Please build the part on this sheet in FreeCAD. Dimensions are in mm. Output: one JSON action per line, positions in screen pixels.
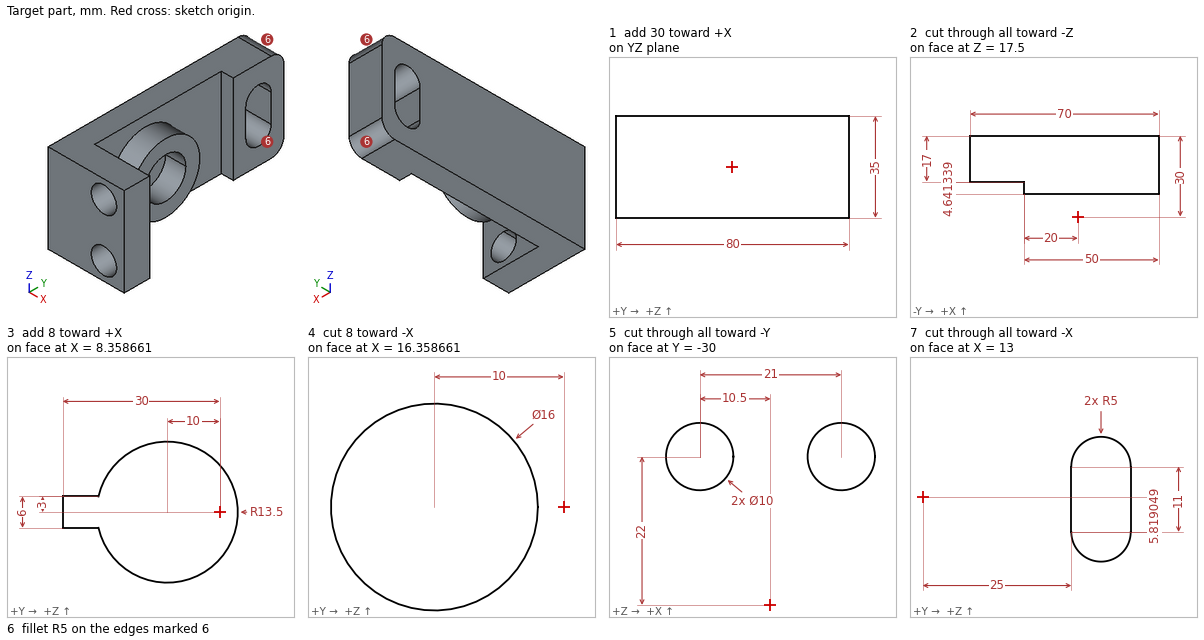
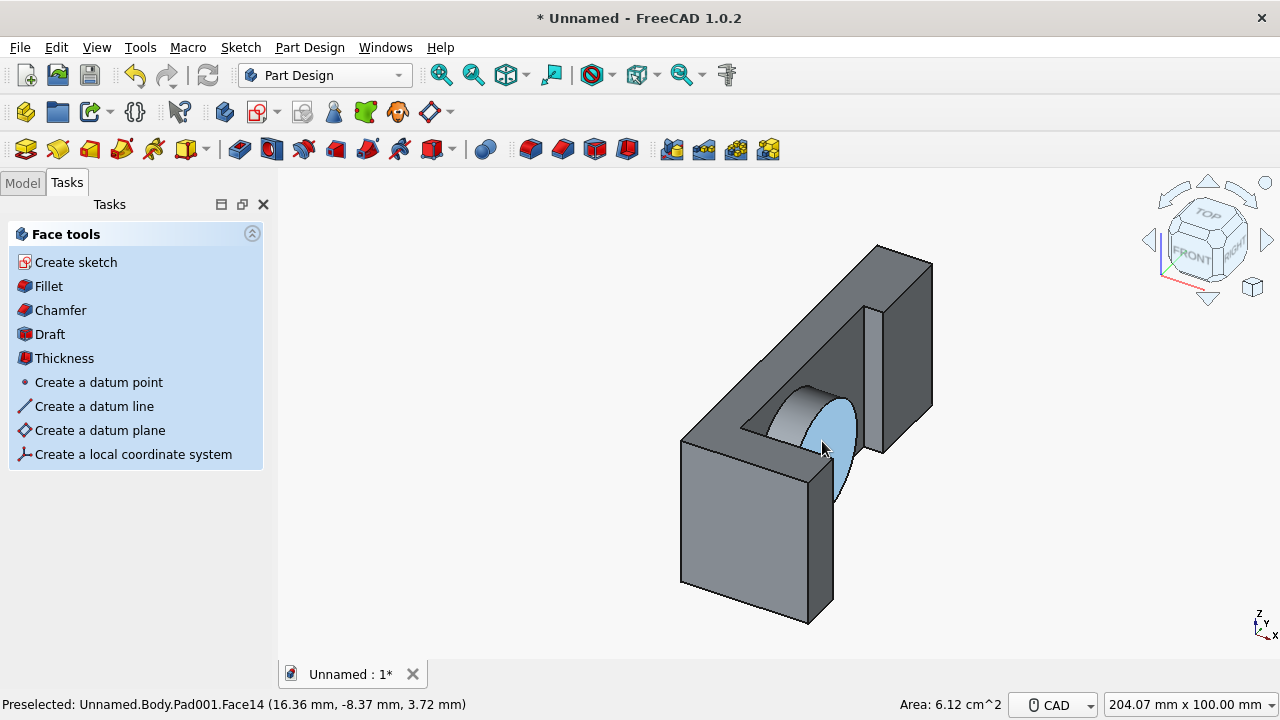
{"action": "left_click", "coordinate": [258, 112]}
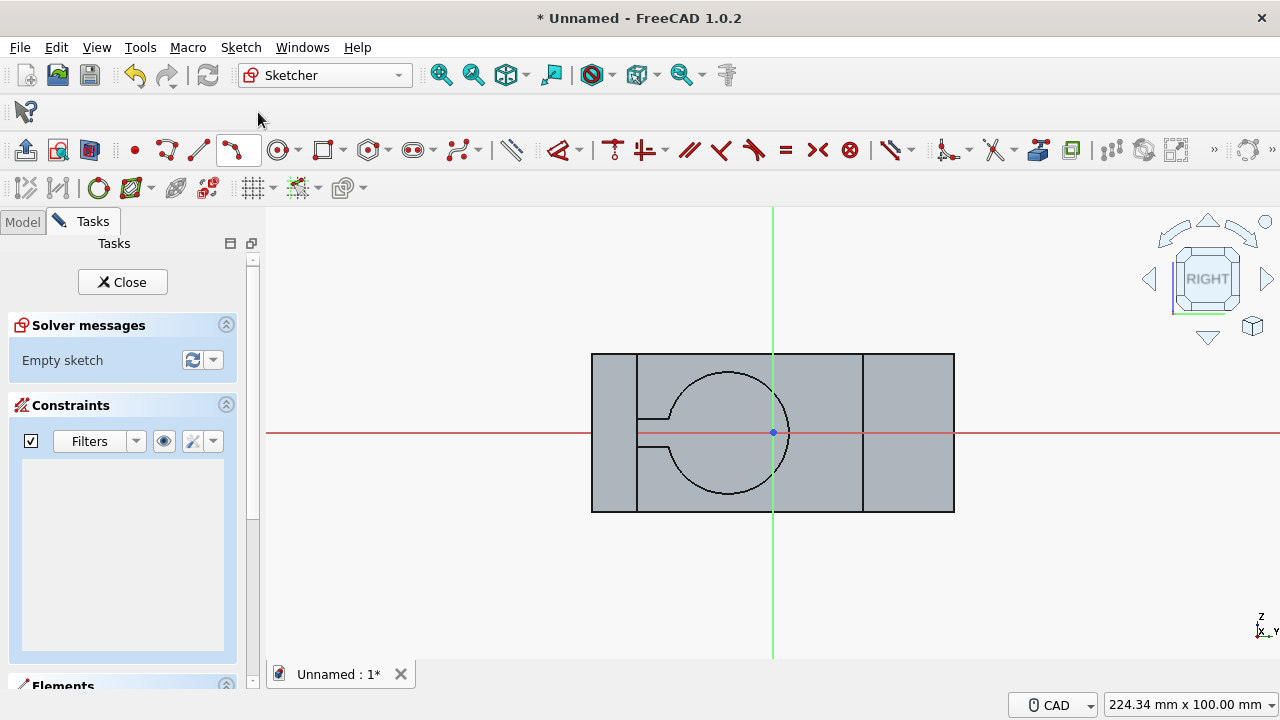
{"action": "left_click", "coordinate": [90, 150]}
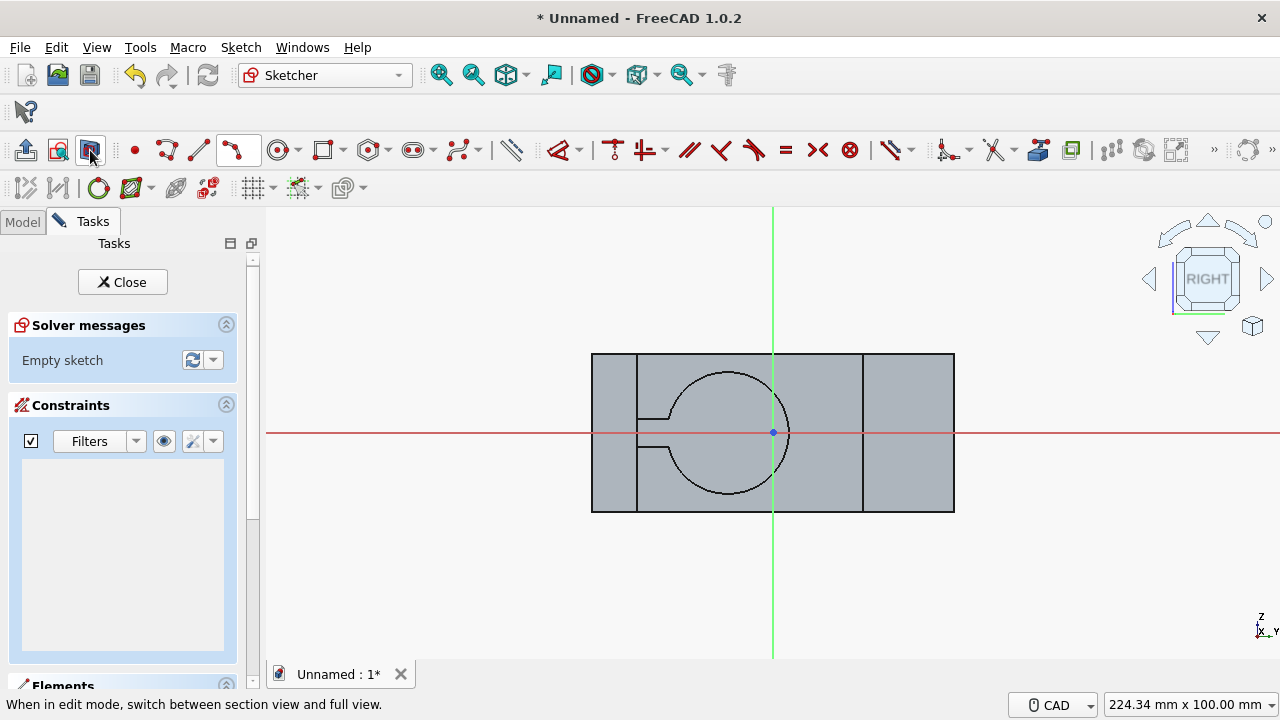
{"action": "scroll", "coordinate": [741, 433], "scroll_direction": "up", "scroll_amount": 7}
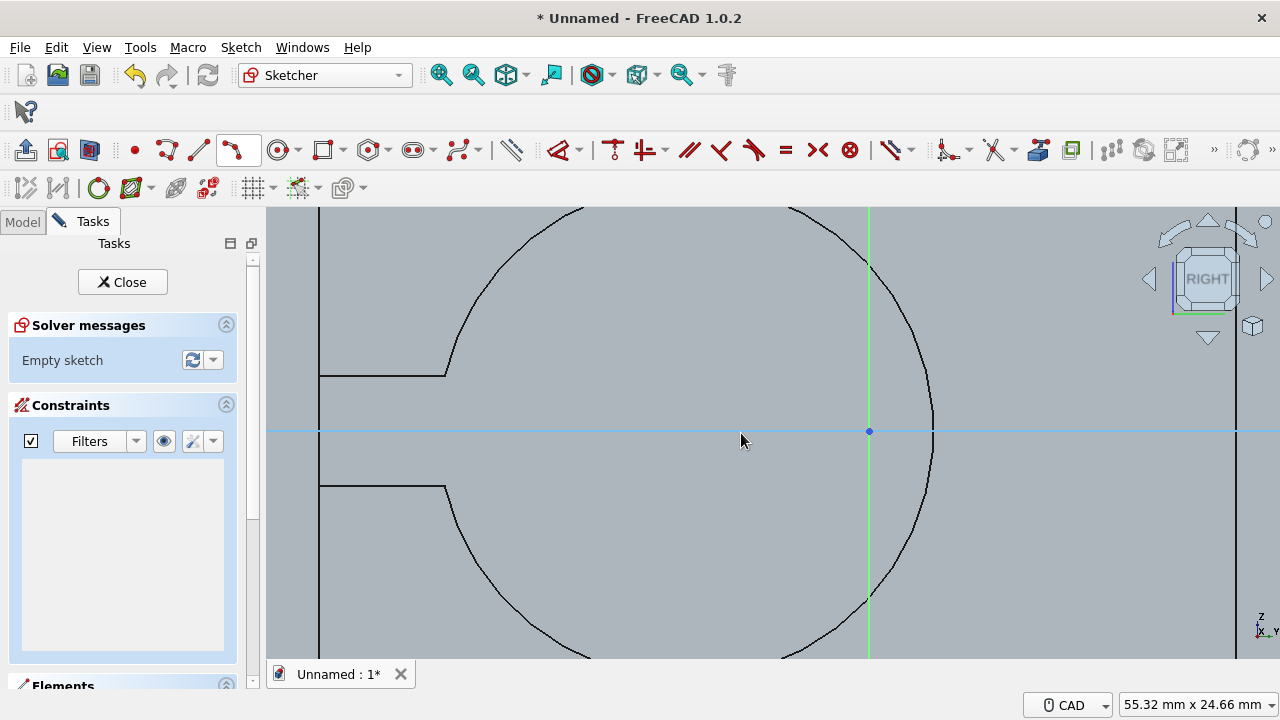
{"action": "left_click", "coordinate": [278, 150]}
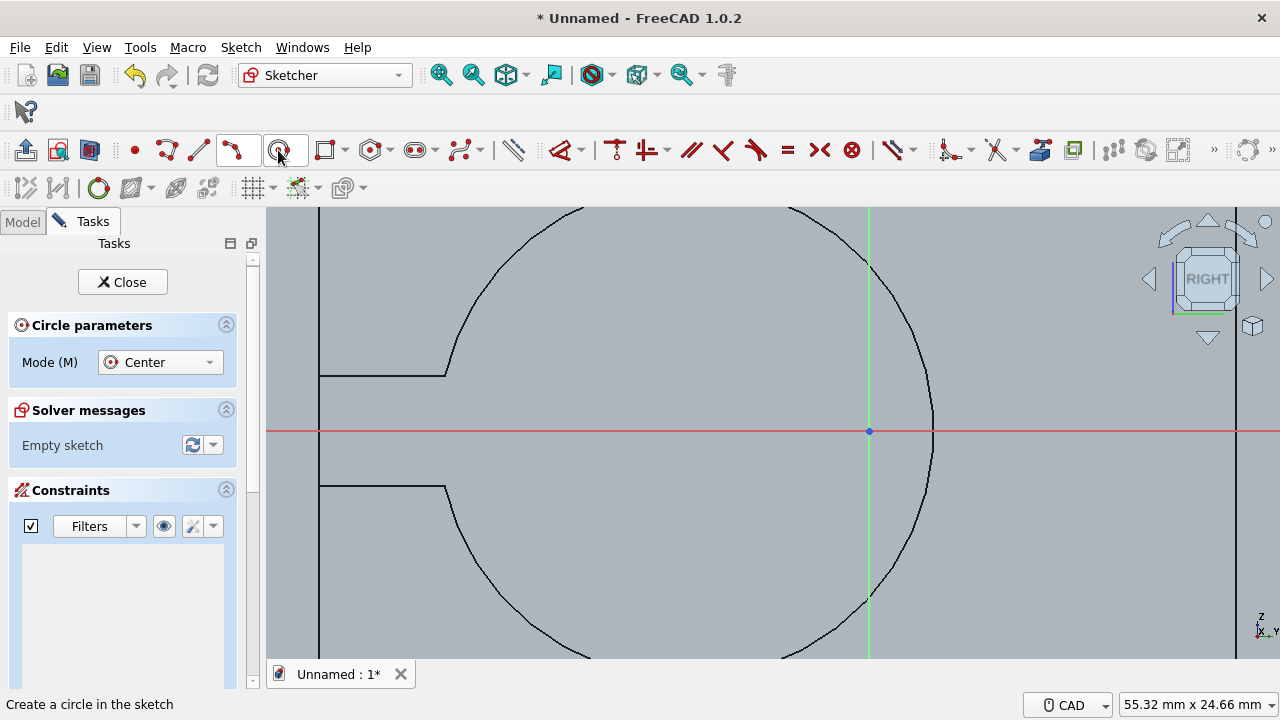
{"action": "left_click", "coordinate": [686, 431]}
{"action": "left_click", "coordinate": [790, 328]}
{"action": "key", "text": "Escape"}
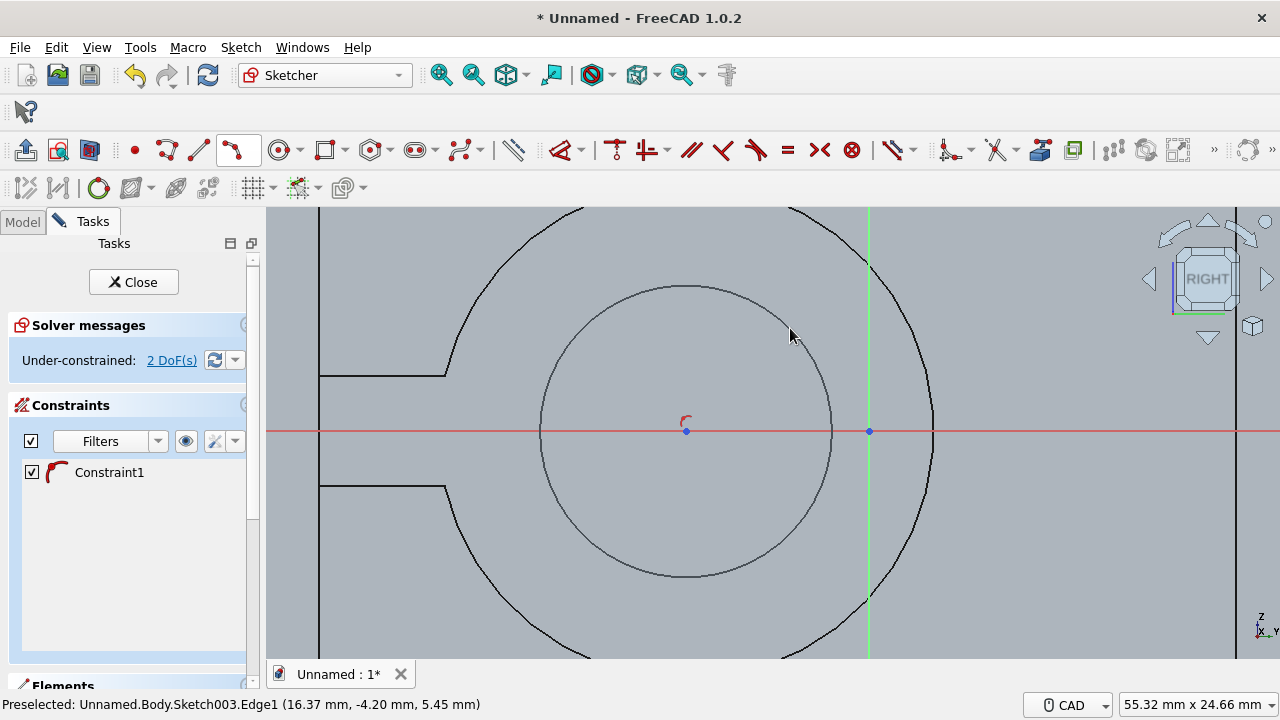
{"action": "left_click", "coordinate": [560, 150]}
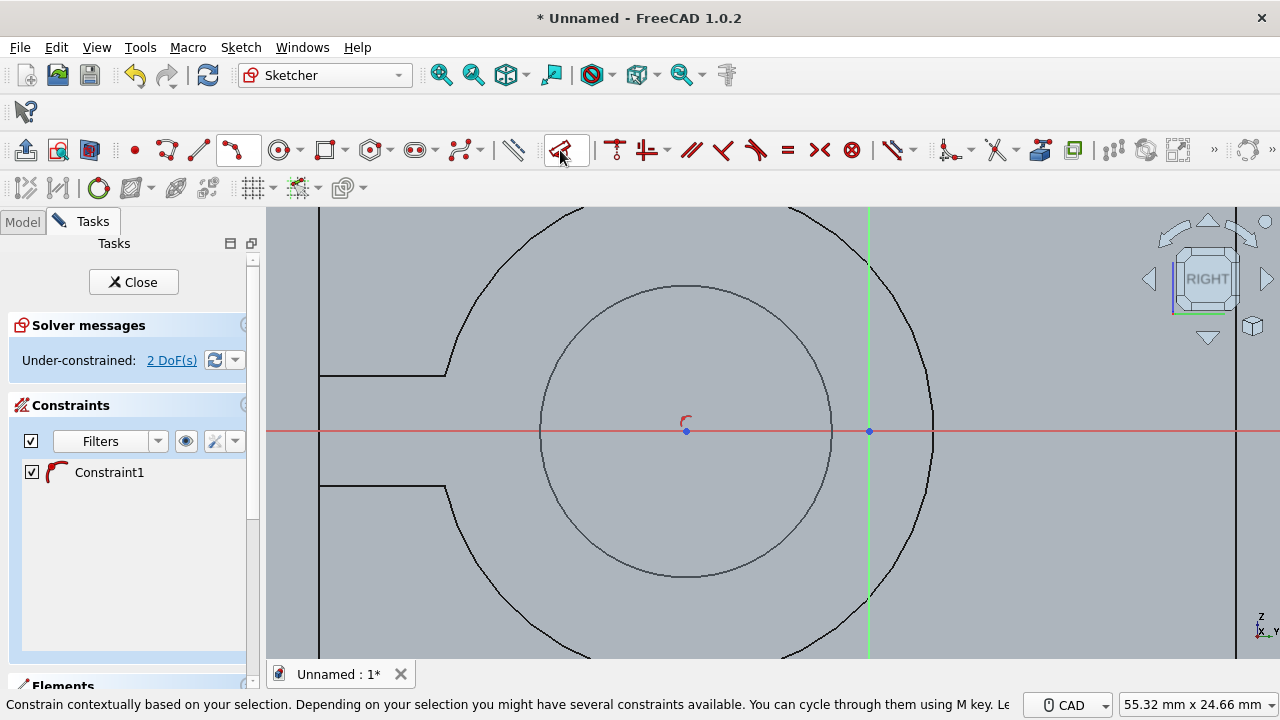
{"action": "left_click", "coordinate": [789, 328]}
{"action": "left_click", "coordinate": [812, 305]}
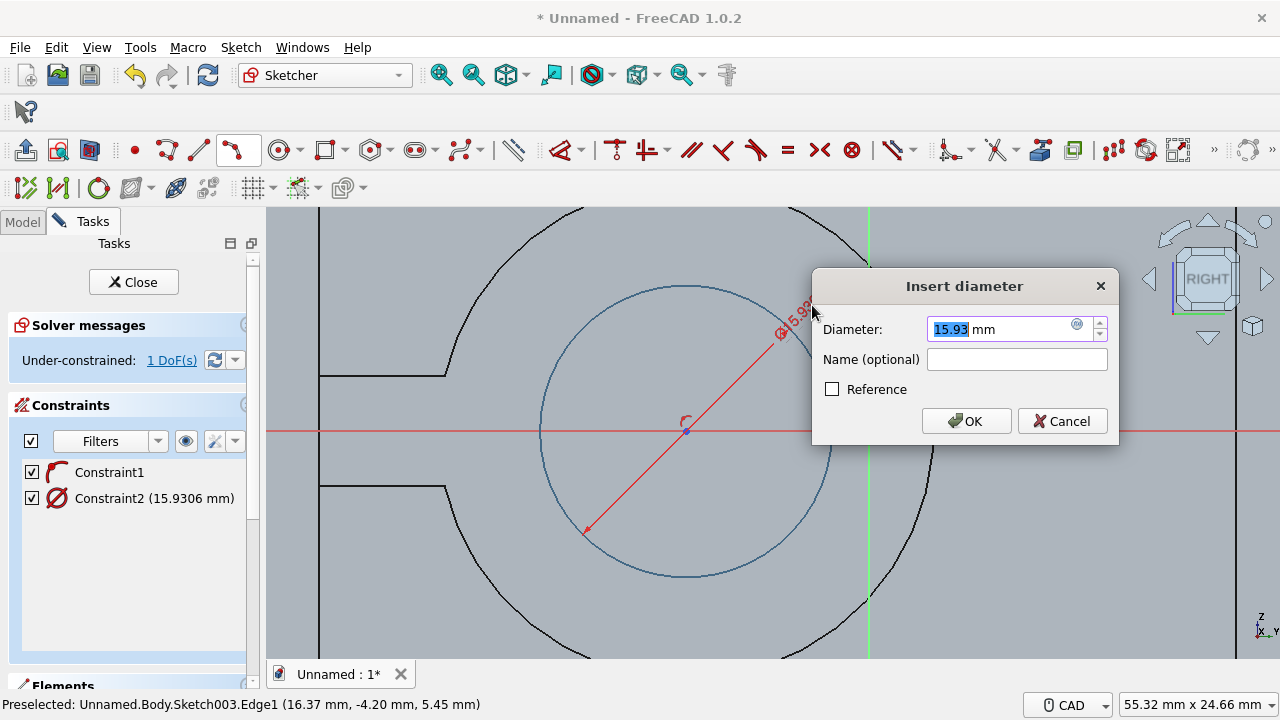
{"action": "type", "text": "16"}
{"action": "key", "text": "Return"}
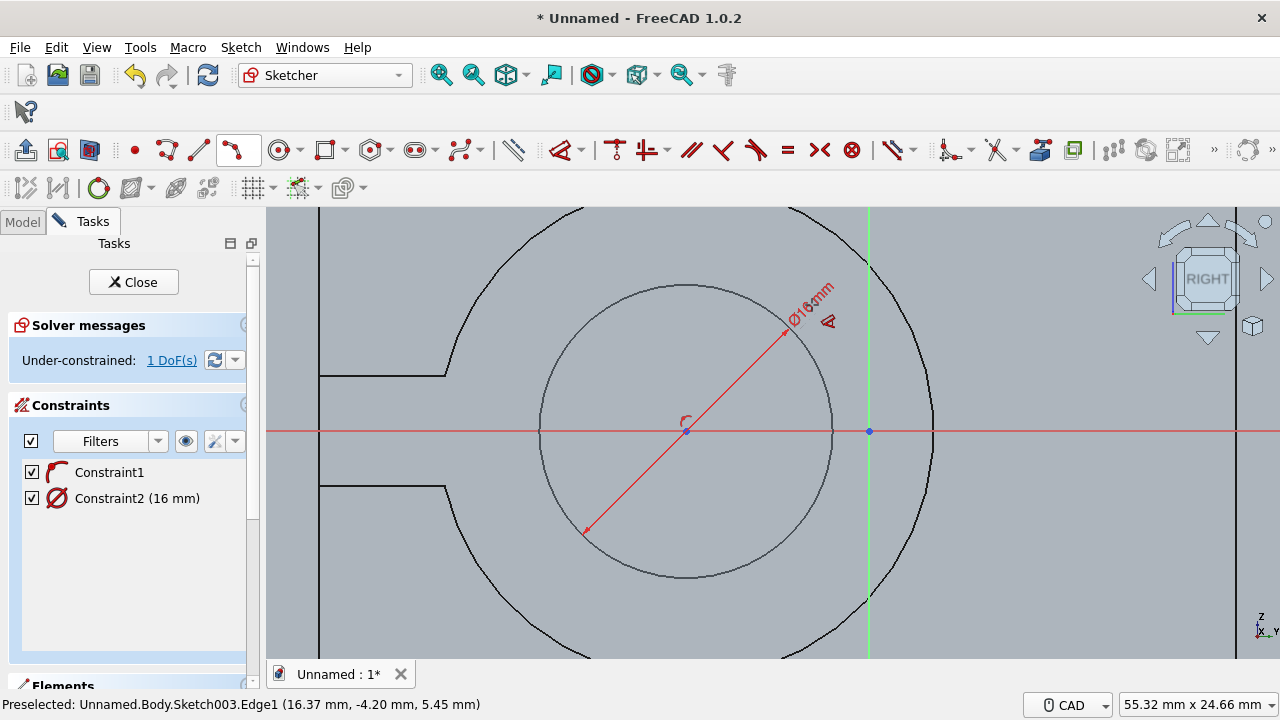
{"action": "left_click", "coordinate": [686, 431]}
{"action": "left_click", "coordinate": [778, 465]}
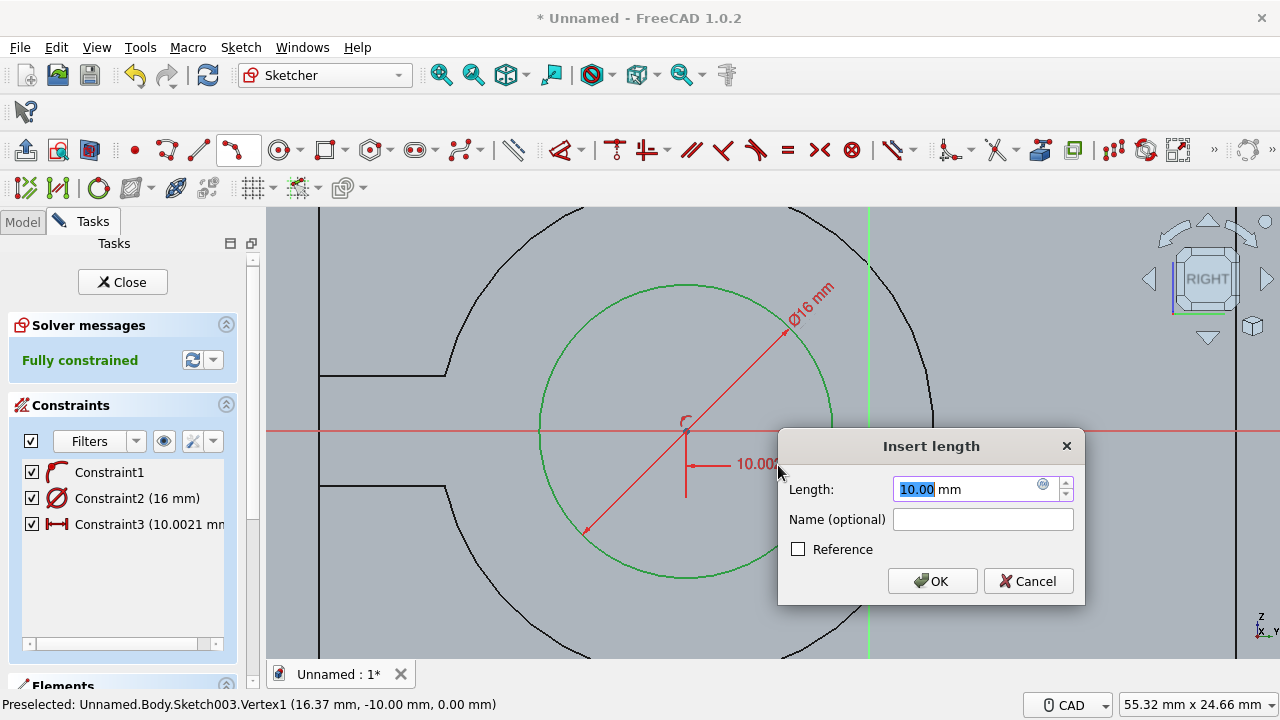
{"action": "type", "text": "10"}
{"action": "key", "text": "Return"}
{"action": "key", "text": "Escape"}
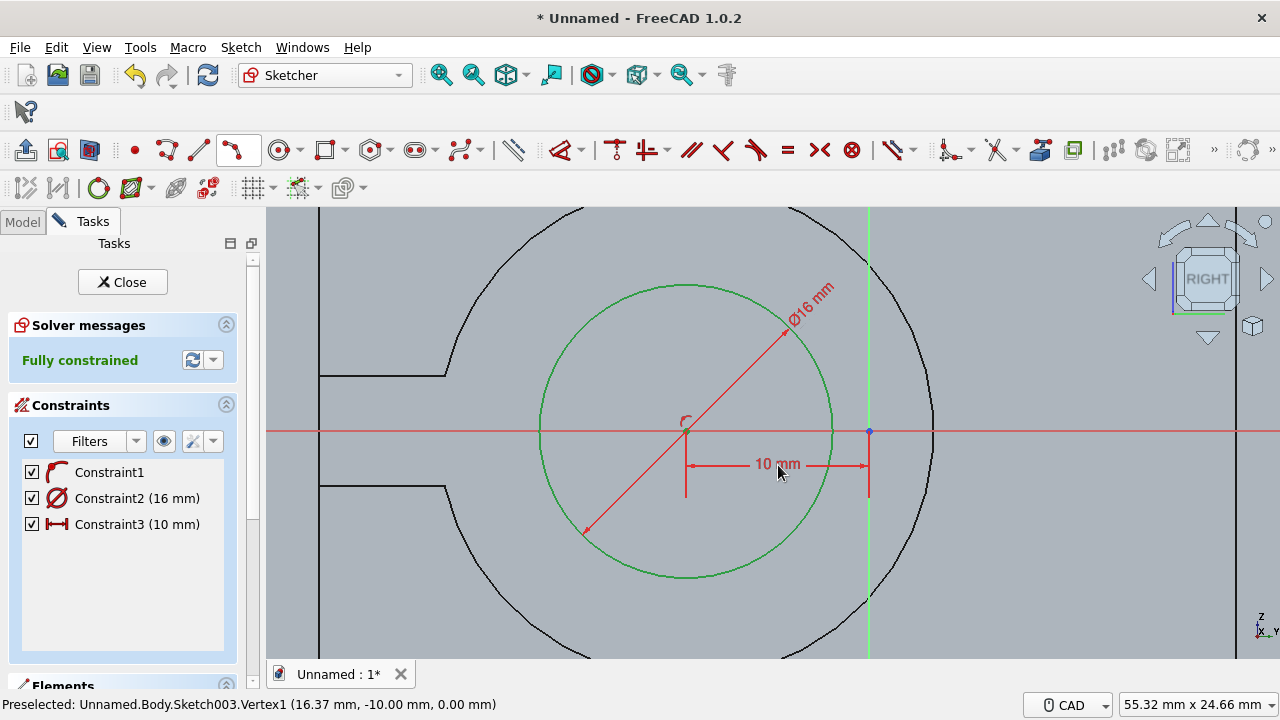
{"action": "left_click", "coordinate": [123, 282]}